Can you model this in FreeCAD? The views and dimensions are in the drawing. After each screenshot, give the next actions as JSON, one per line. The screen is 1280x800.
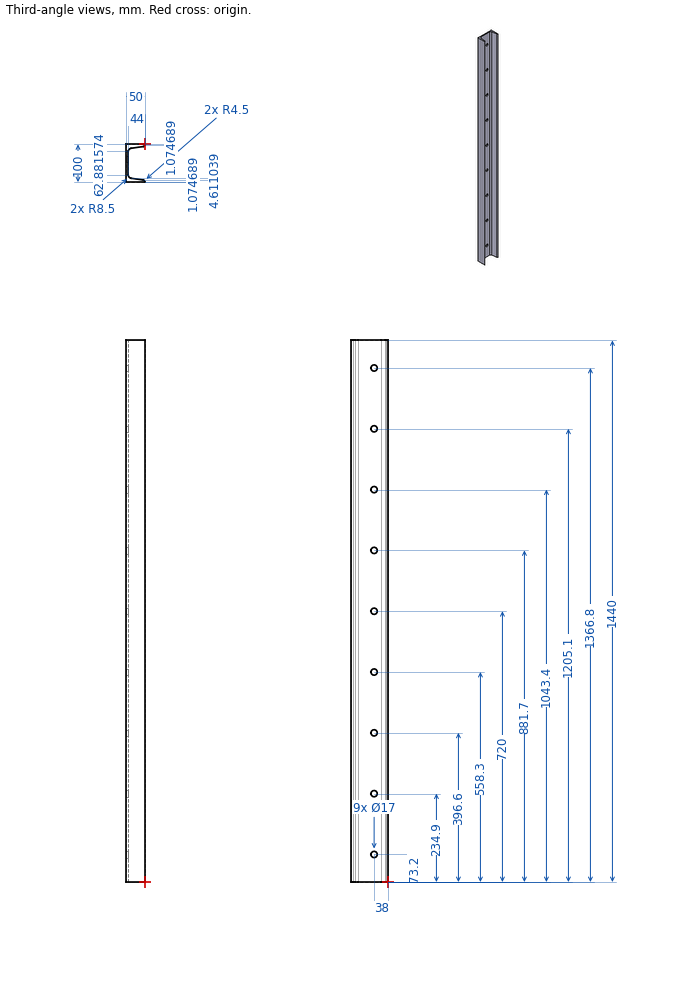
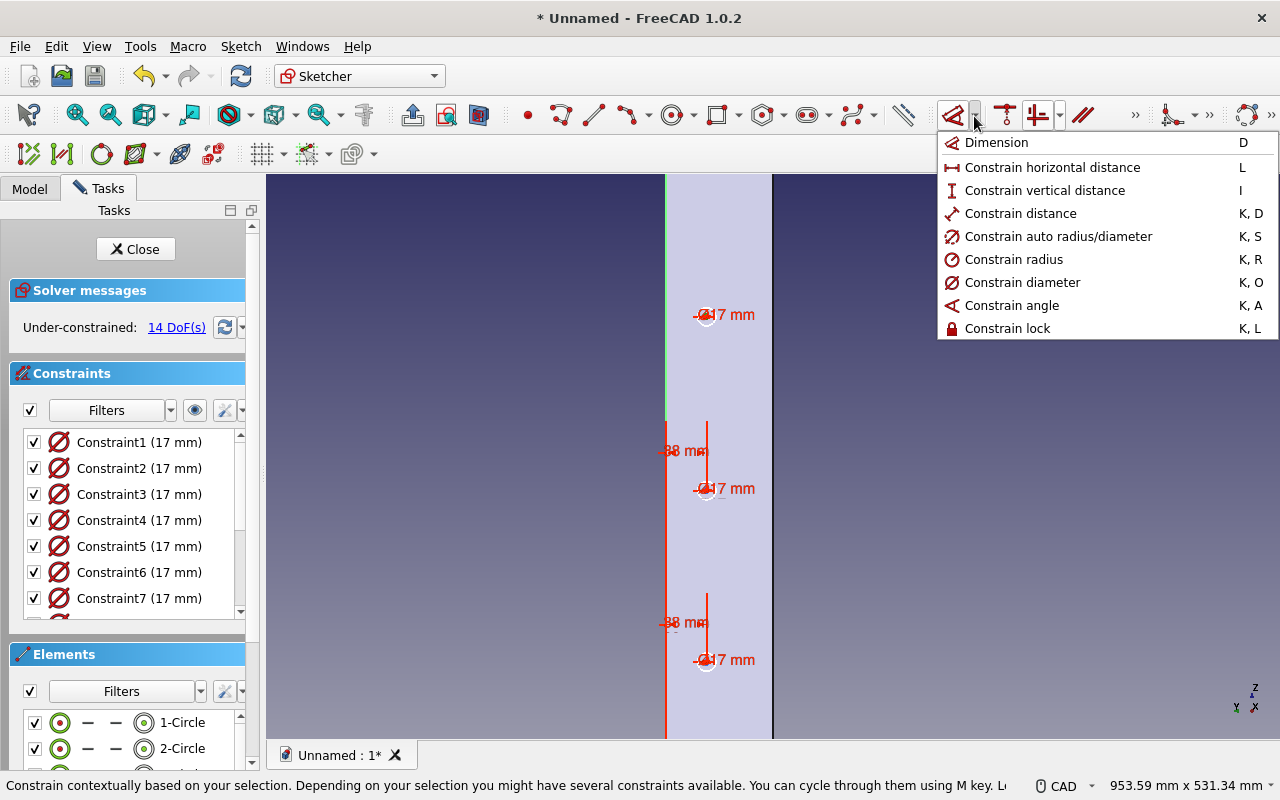
{"action": "left_click", "coordinate": [1108, 168]}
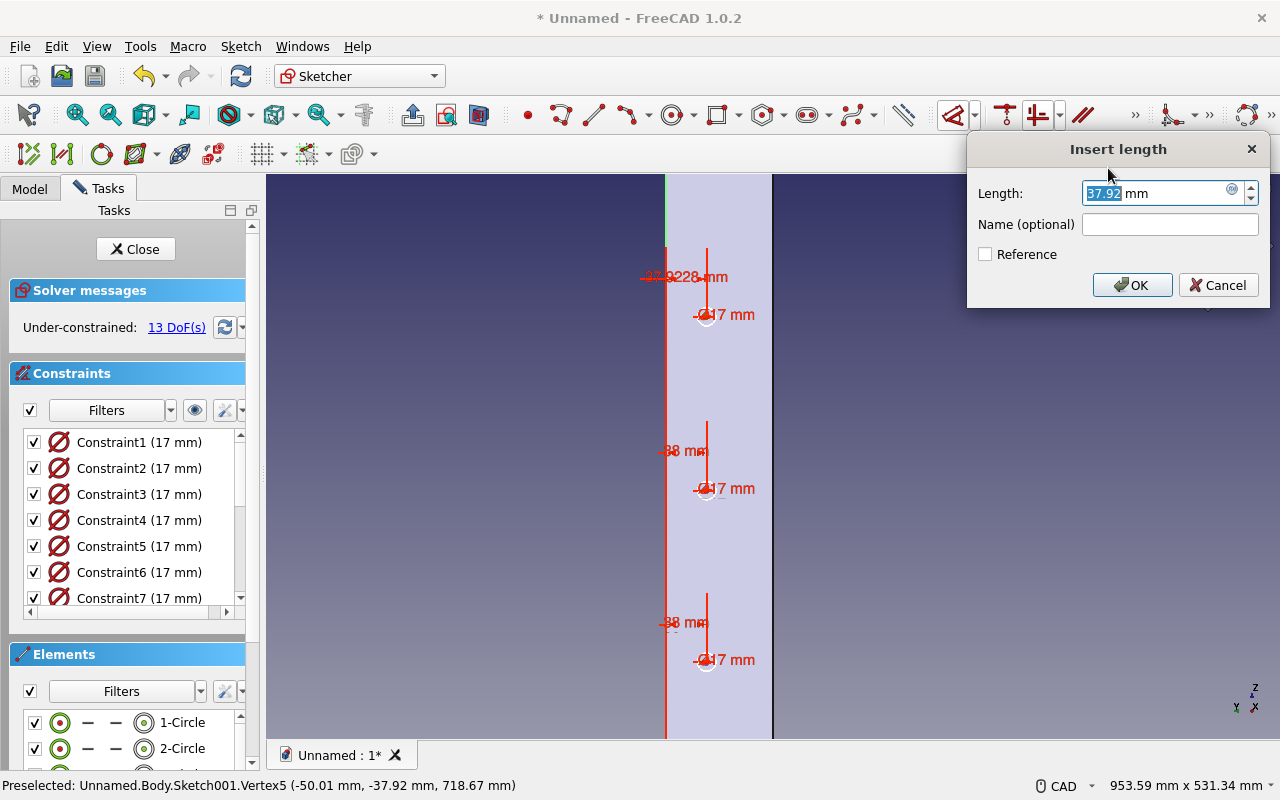
{"action": "type", "text": "38"}
{"action": "key", "text": "Return"}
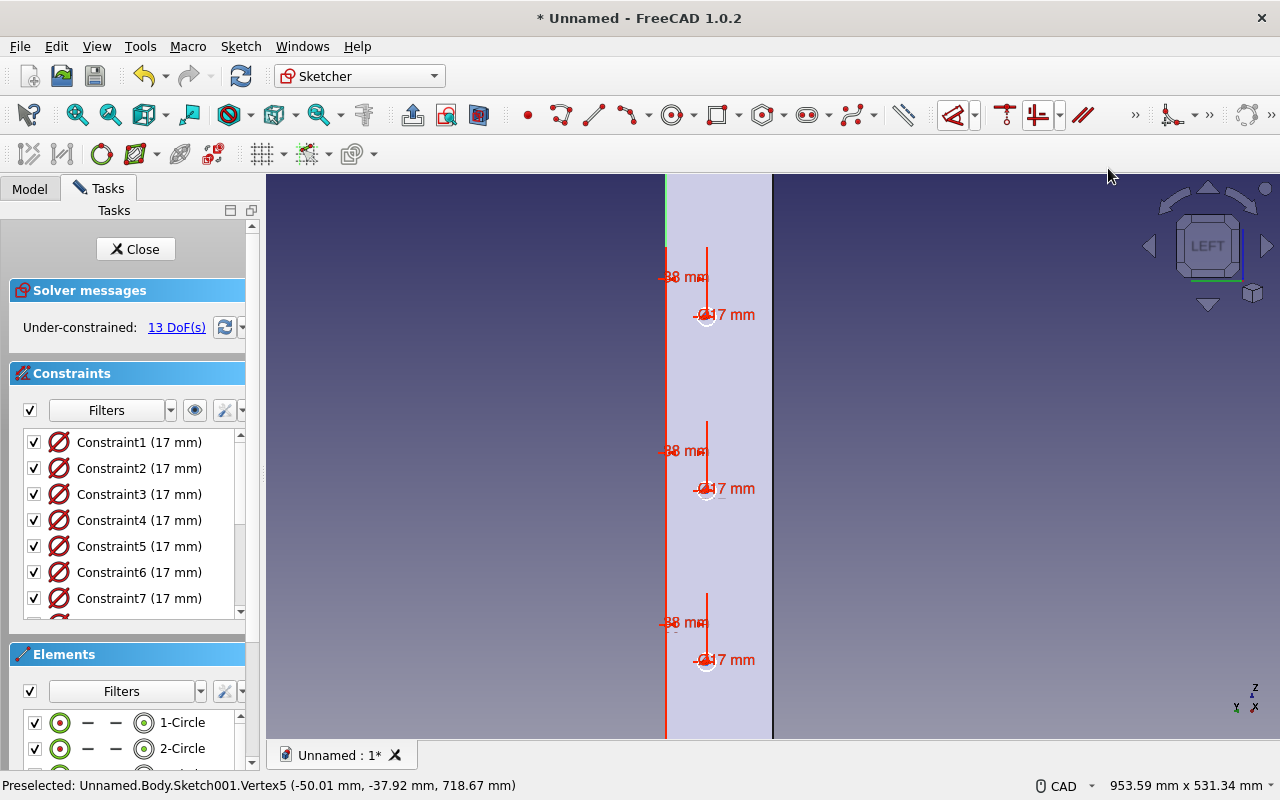
{"action": "scroll", "coordinate": [709, 491], "scroll_direction": "down", "scroll_amount": 7}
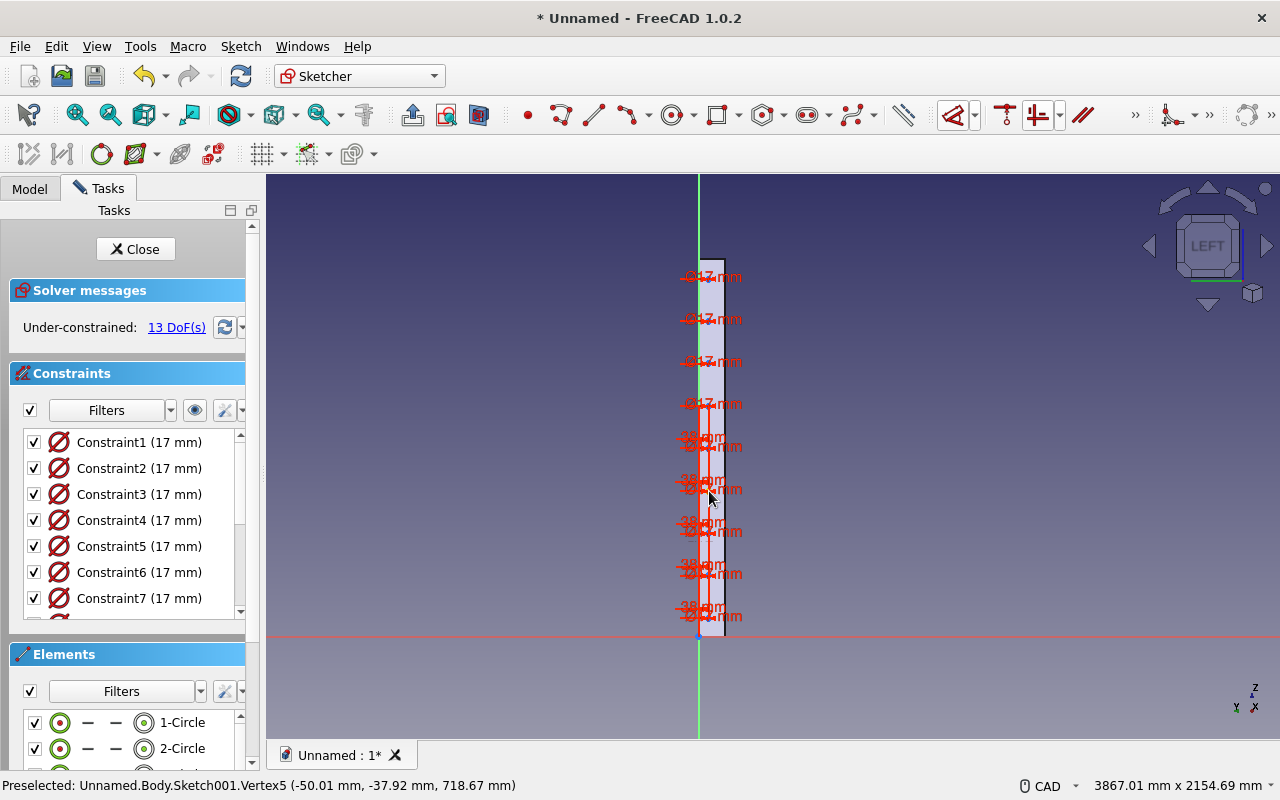
{"action": "scroll", "coordinate": [709, 406], "scroll_direction": "up", "scroll_amount": 7}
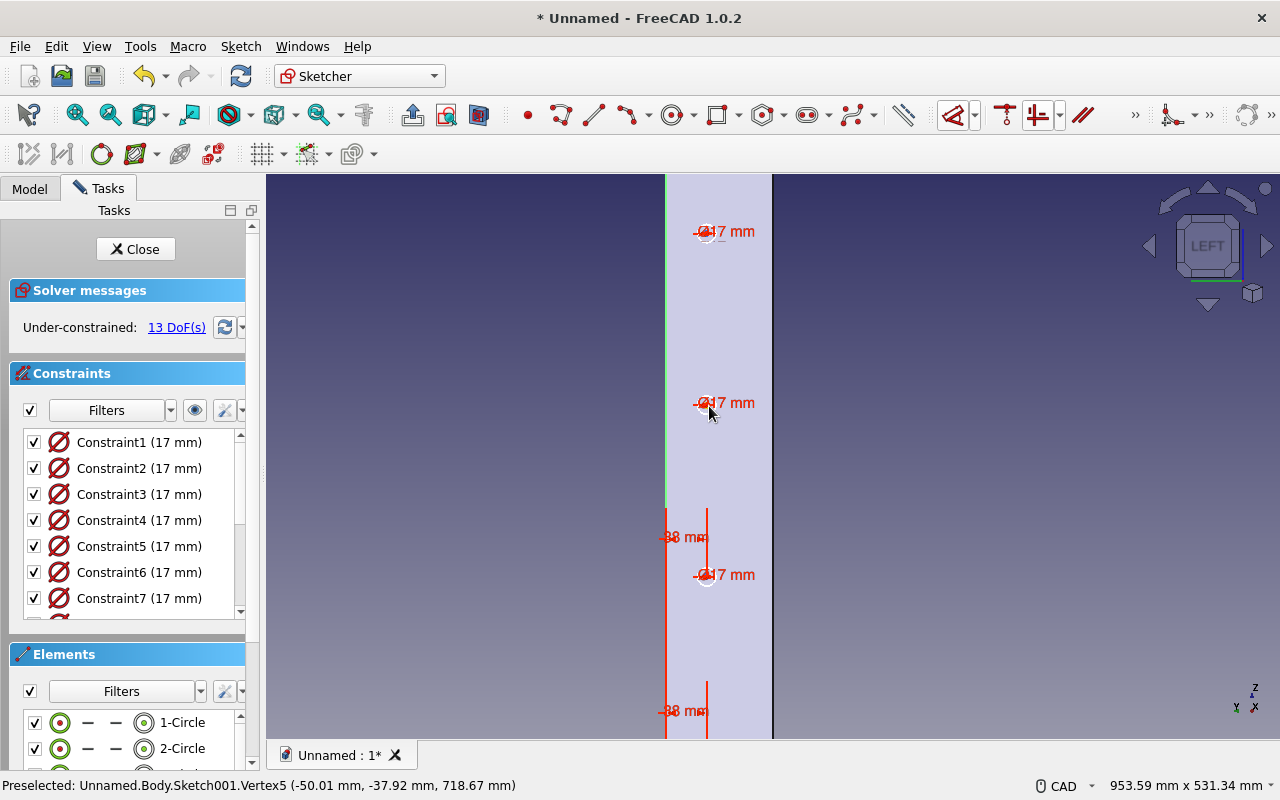
{"action": "left_click", "coordinate": [707, 405]}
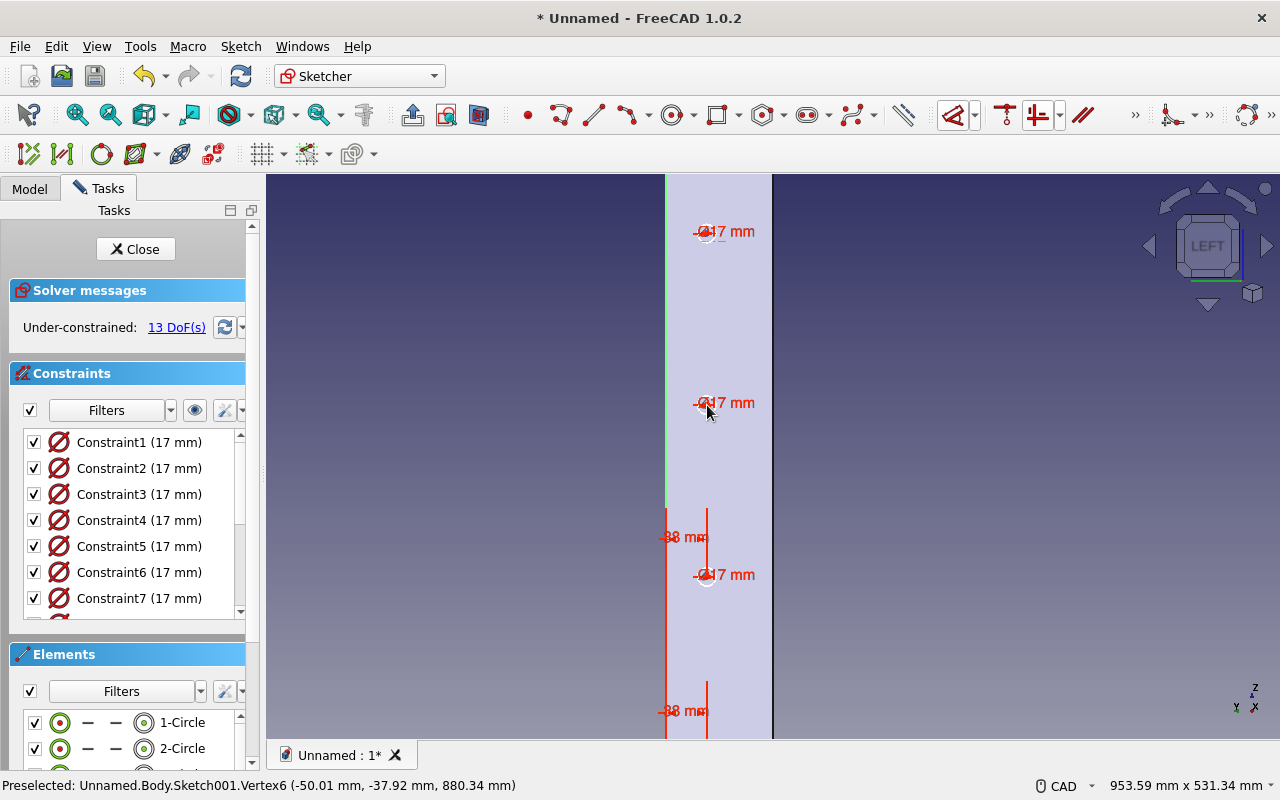
{"action": "key", "text": "l"}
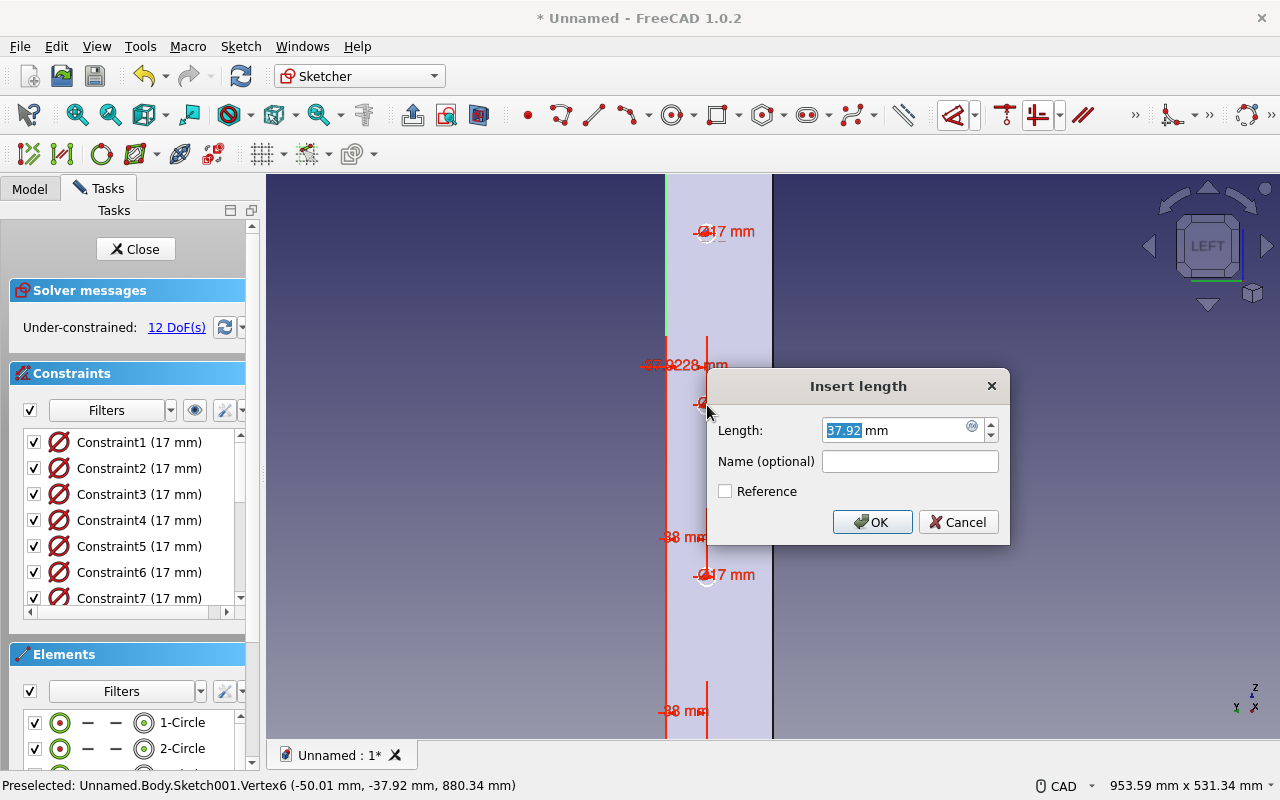
{"action": "type", "text": "38"}
{"action": "key", "text": "Return"}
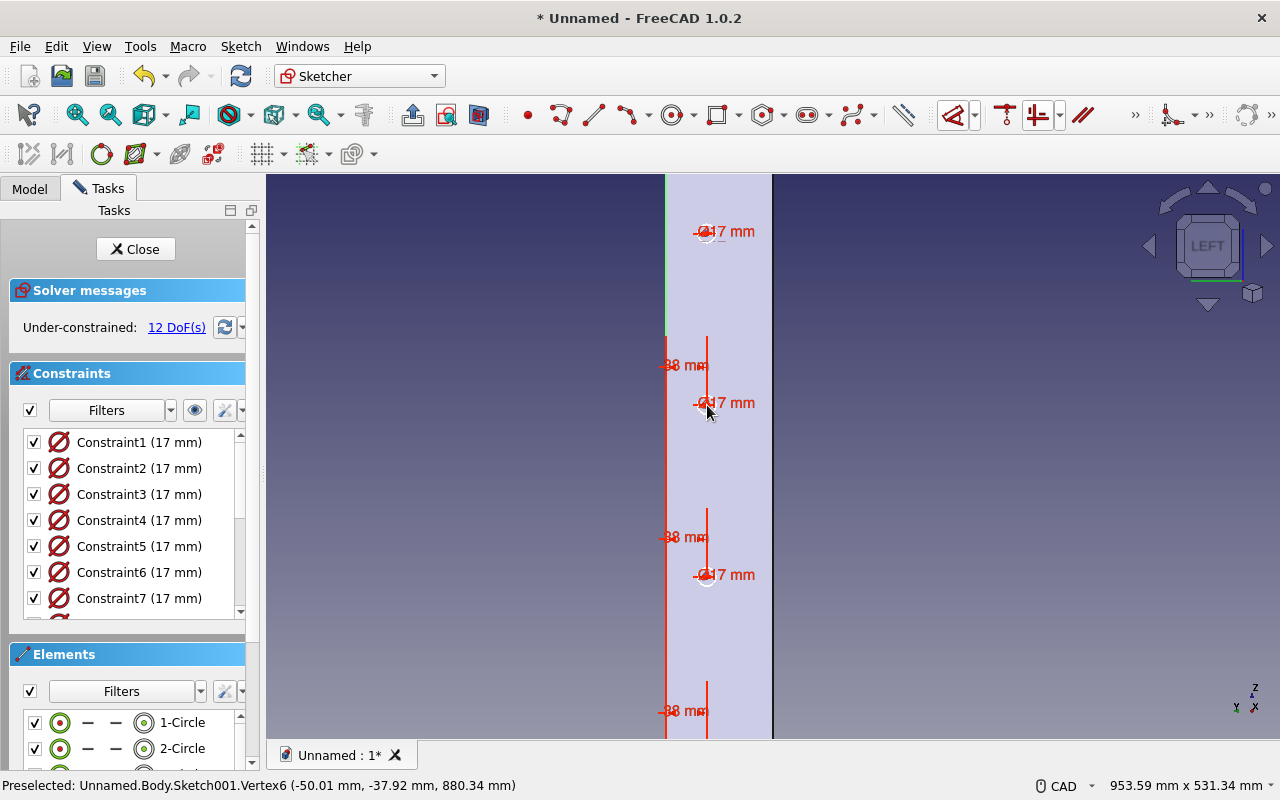
{"action": "left_click", "coordinate": [707, 234]}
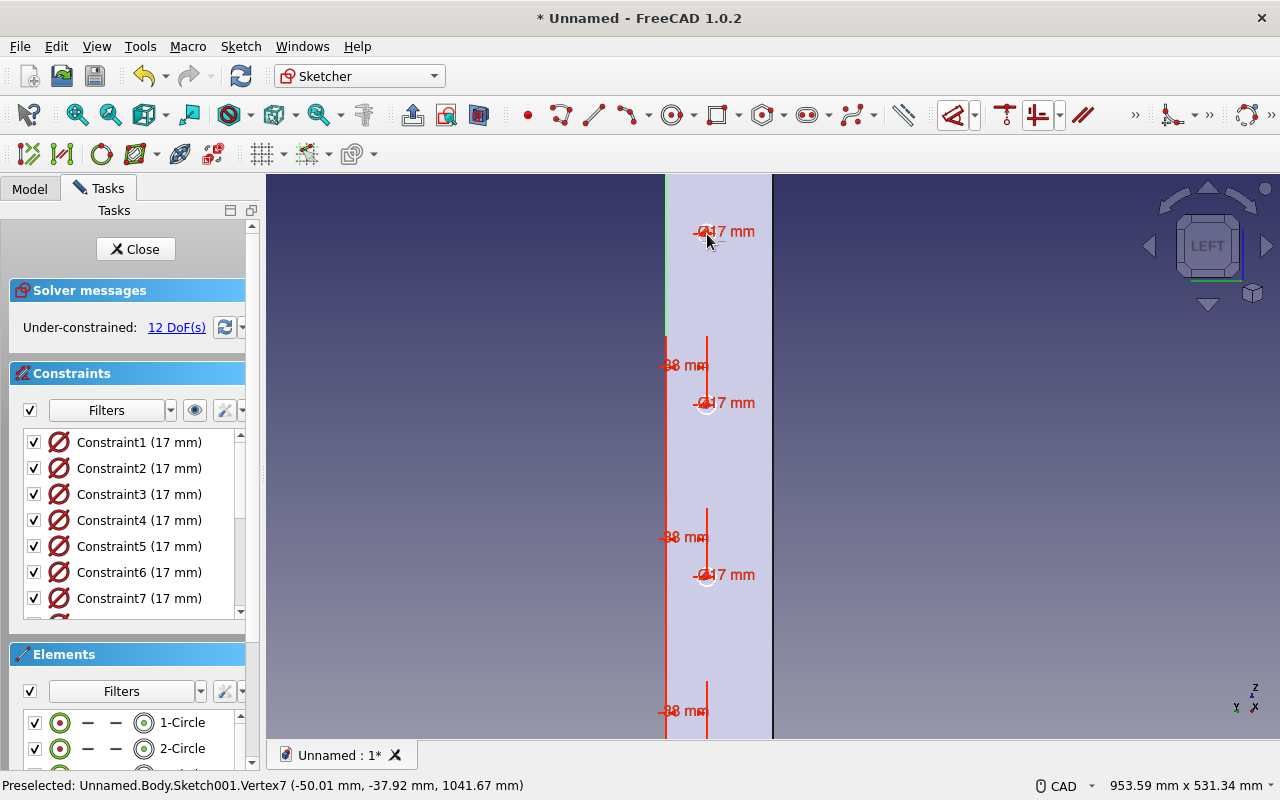
{"action": "left_click", "coordinate": [974, 116]}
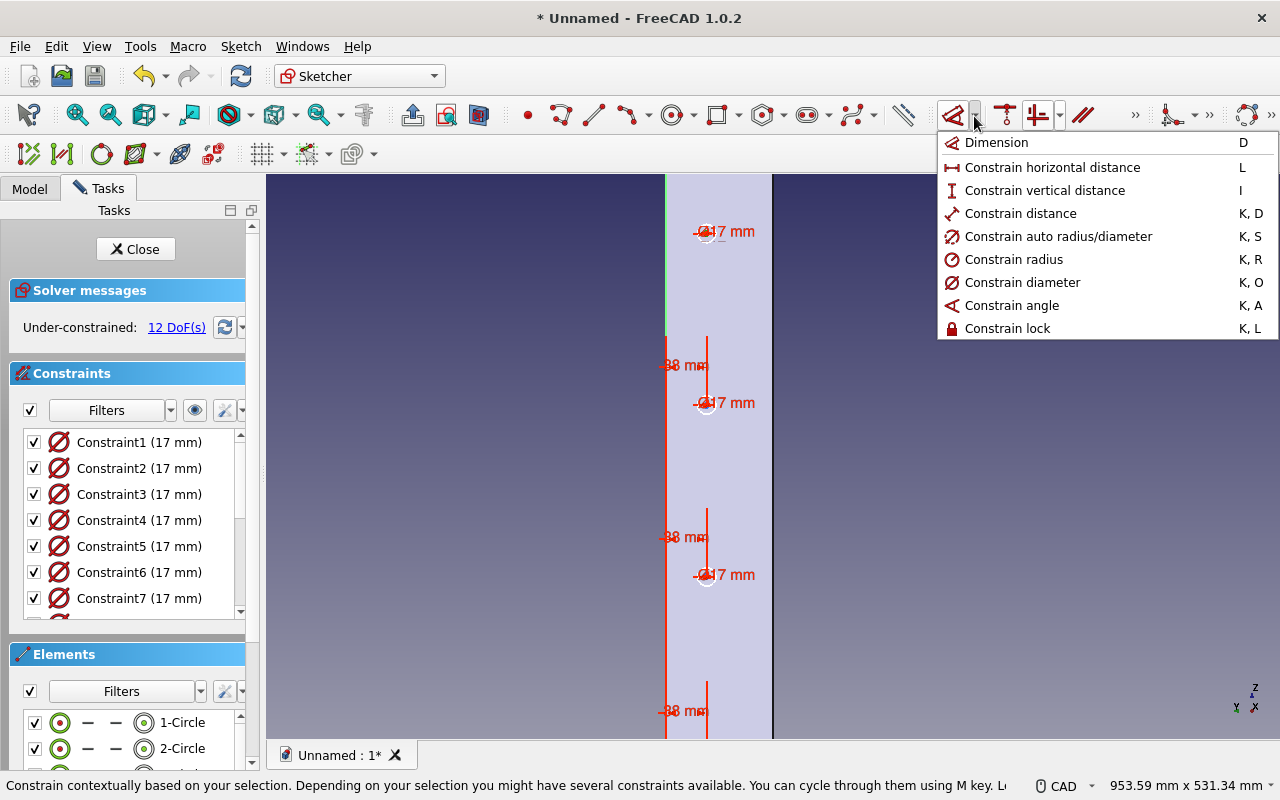
{"action": "left_click", "coordinate": [1108, 168]}